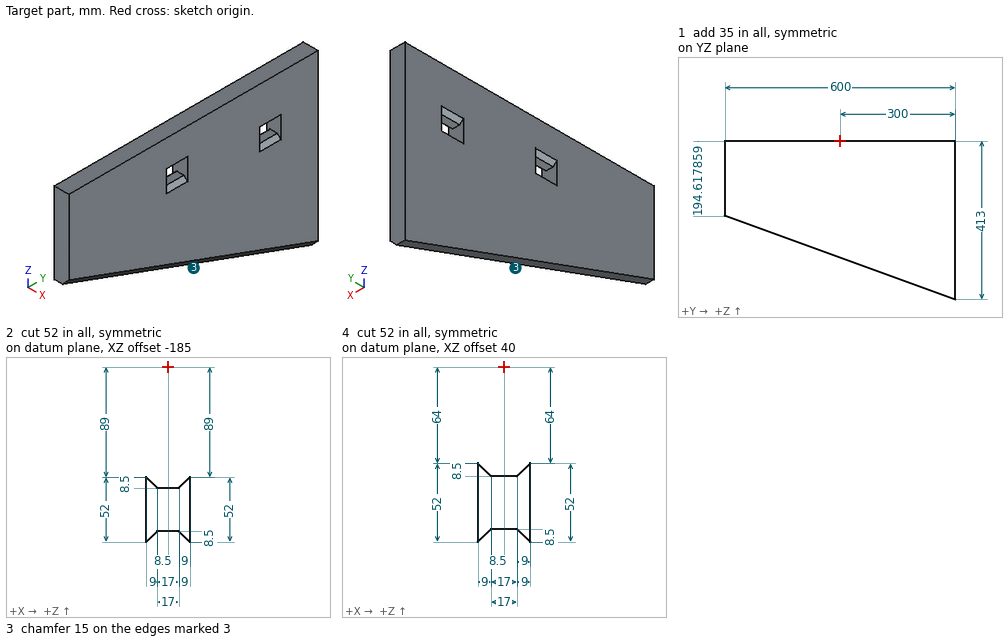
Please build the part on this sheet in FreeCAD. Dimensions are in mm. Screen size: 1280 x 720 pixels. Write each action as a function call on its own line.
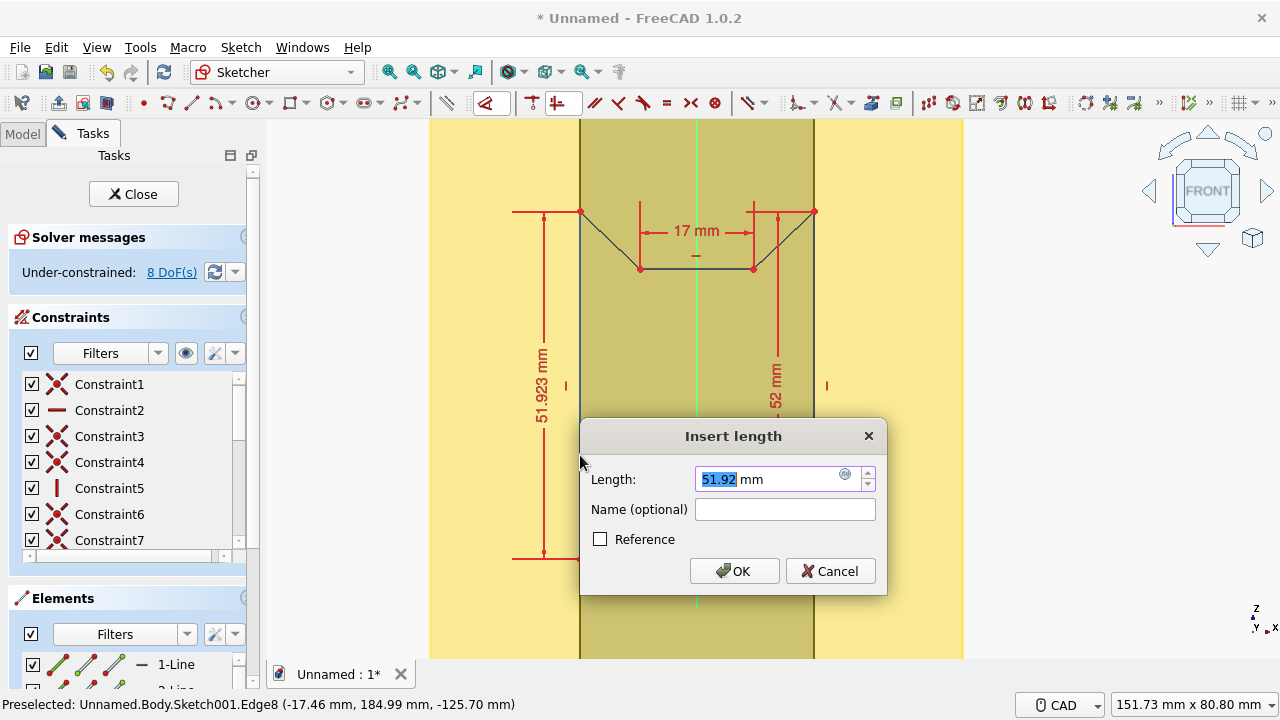
text(52)
key(Return)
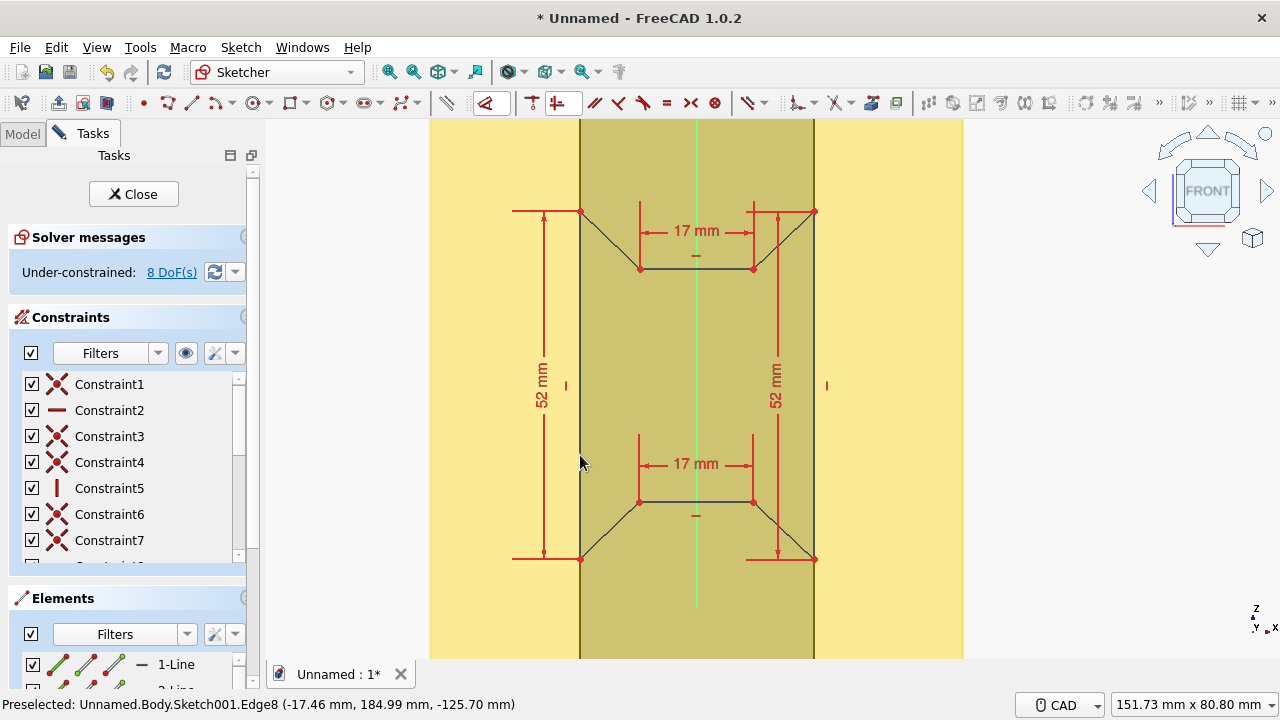
click(598, 229)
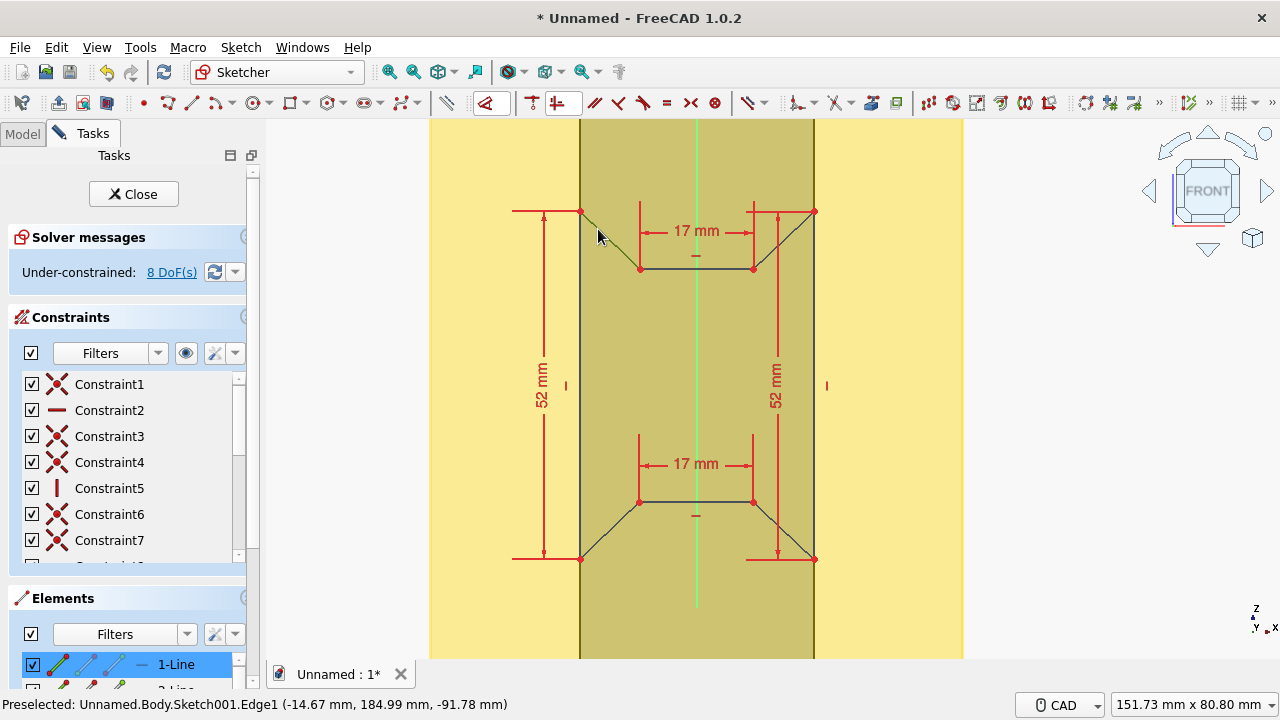
key(l)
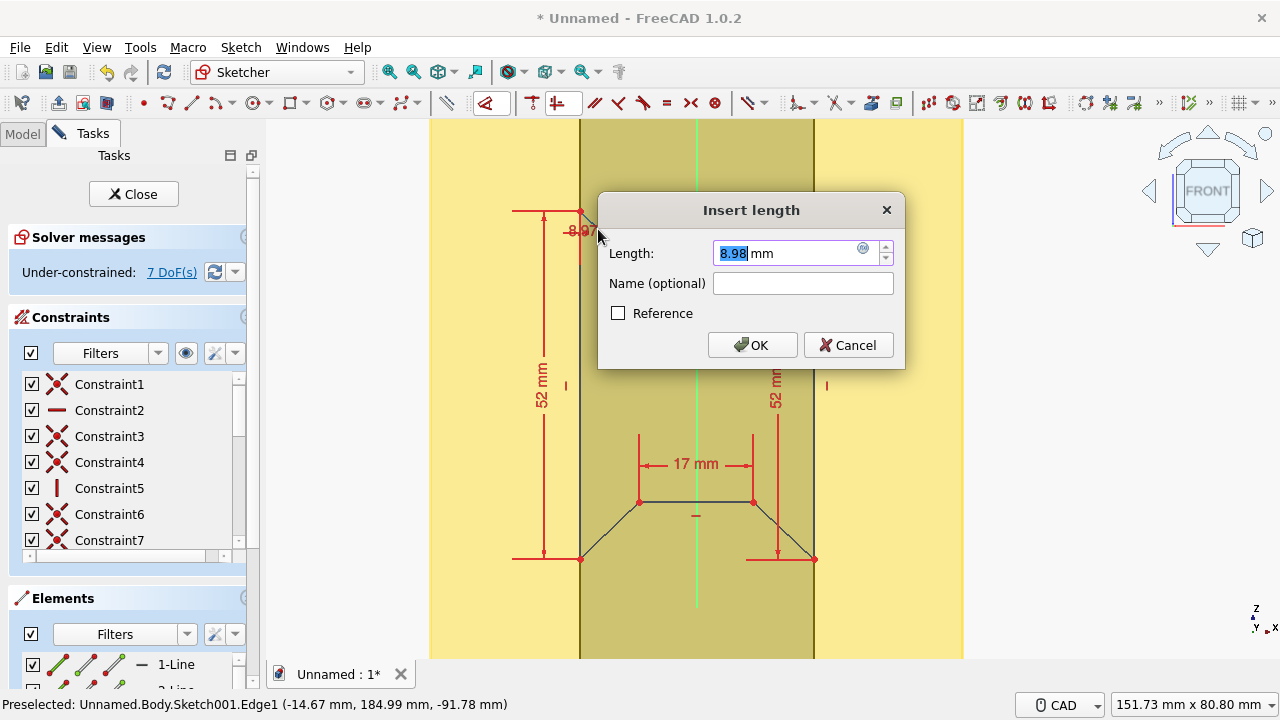
text(9)
key(Return)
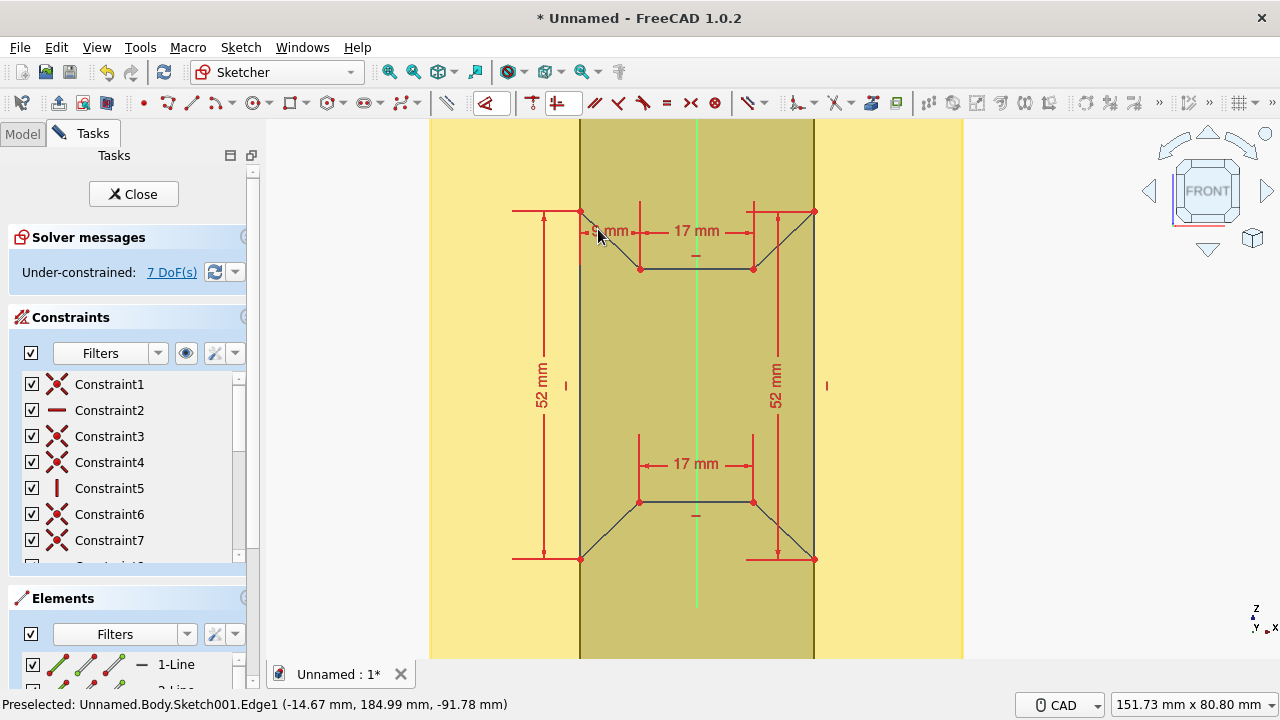
click(772, 252)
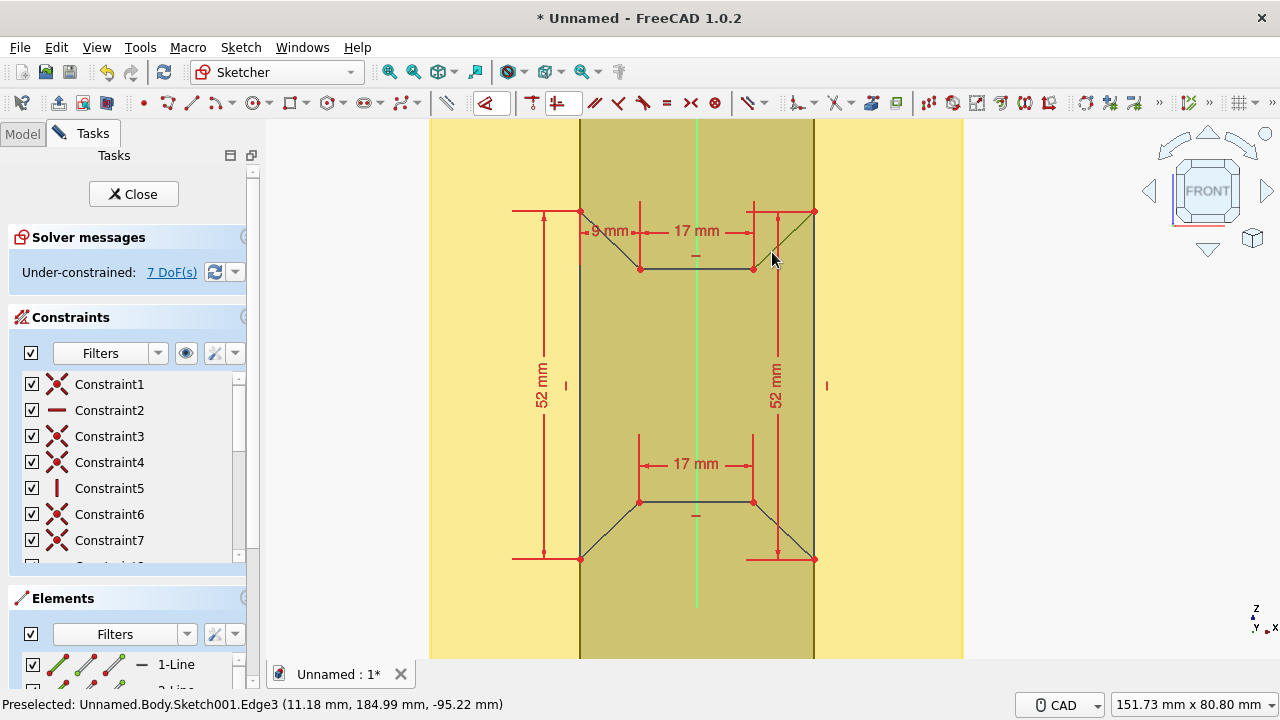
key(l)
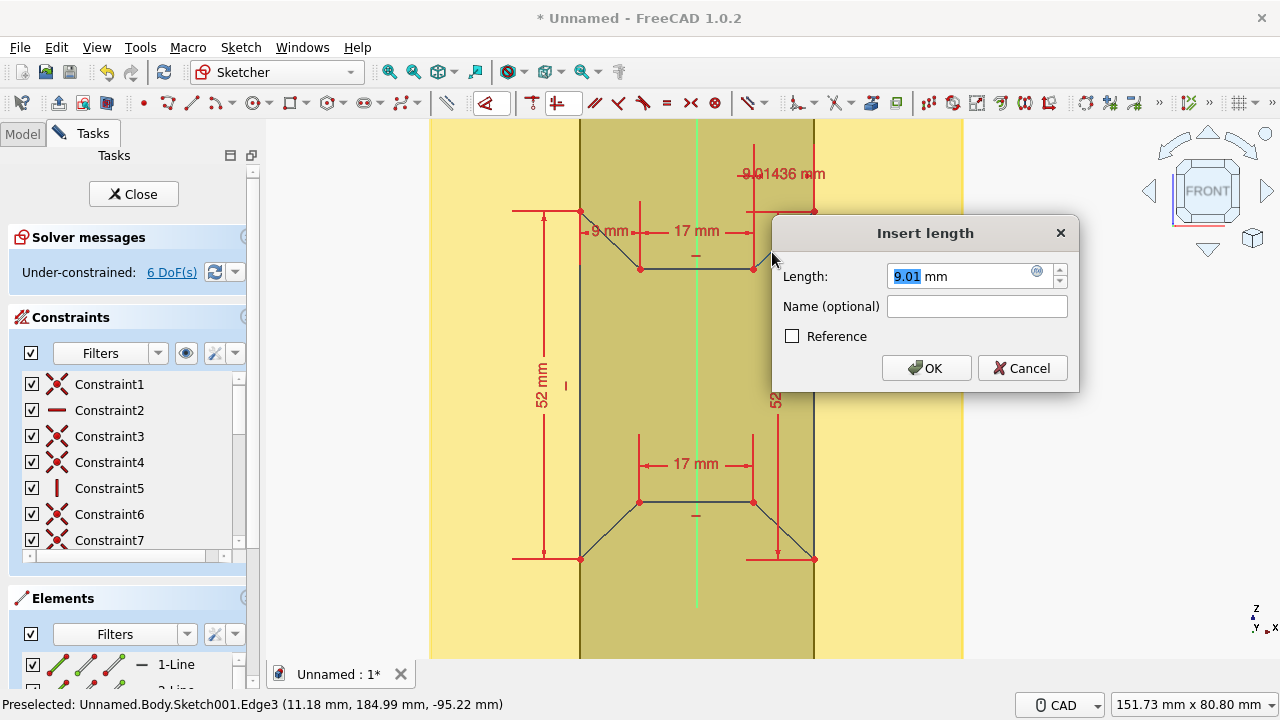
text(9)
key(Return)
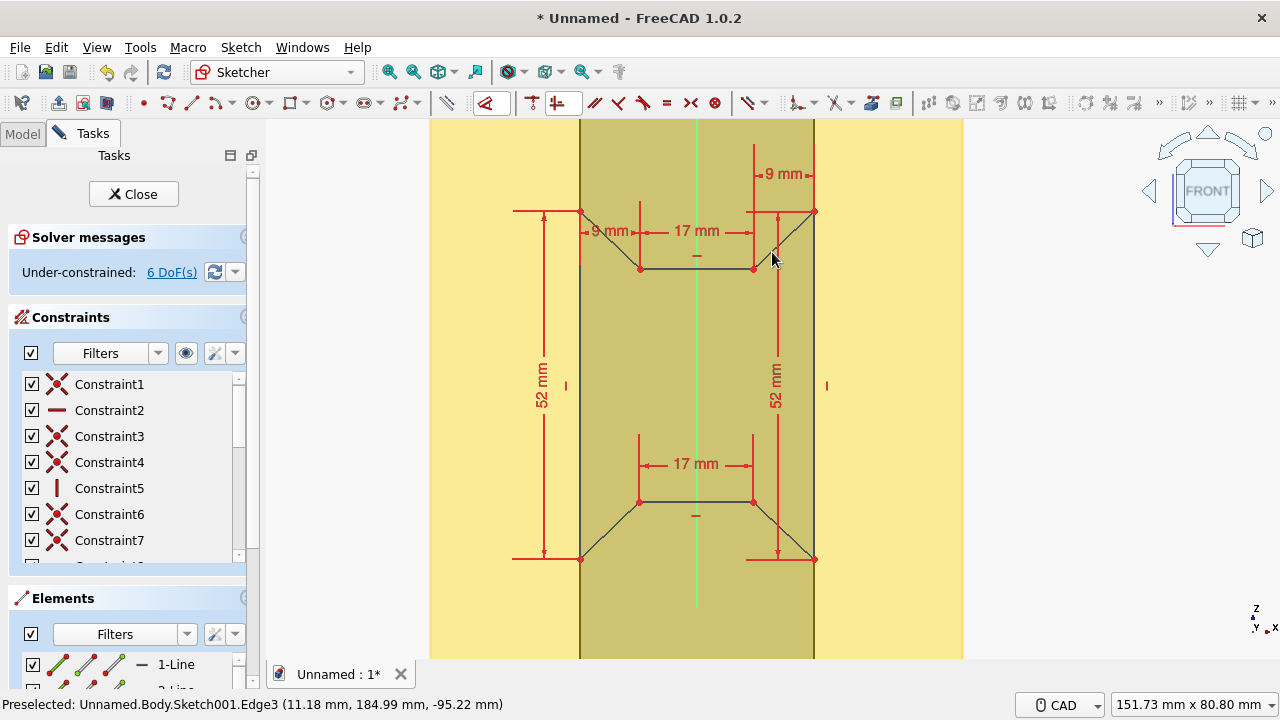
click(796, 542)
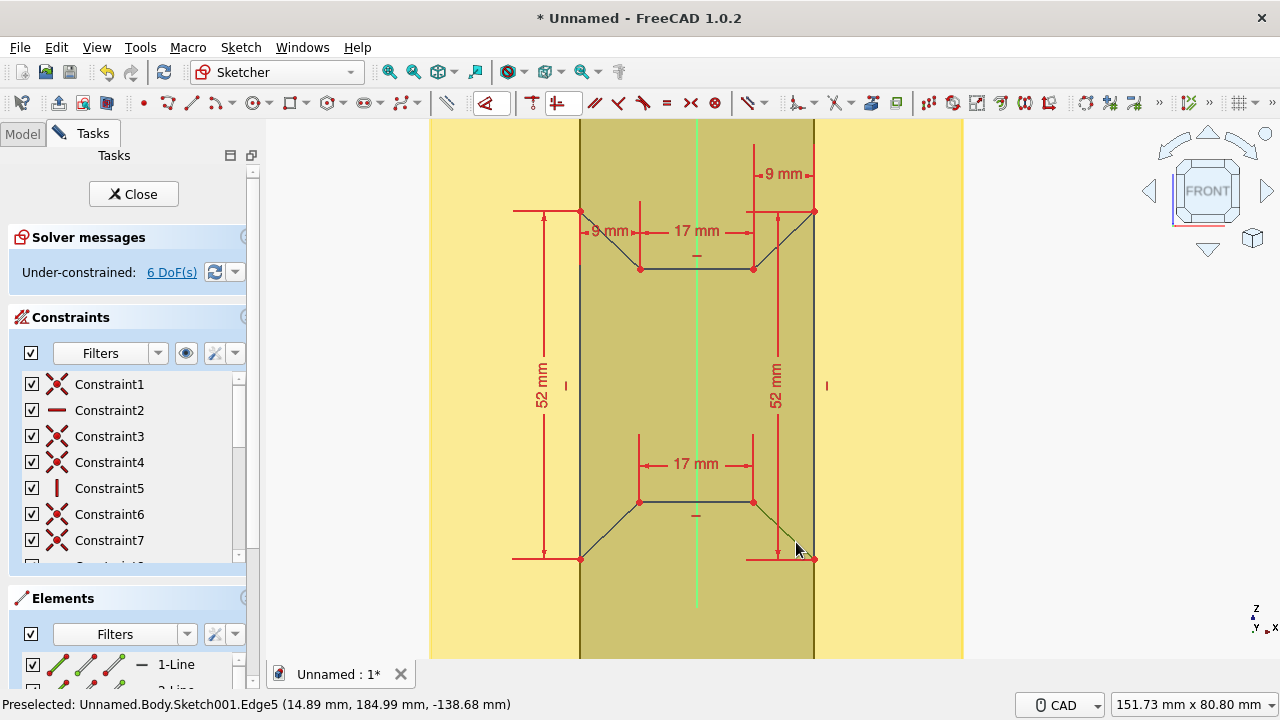
key(l)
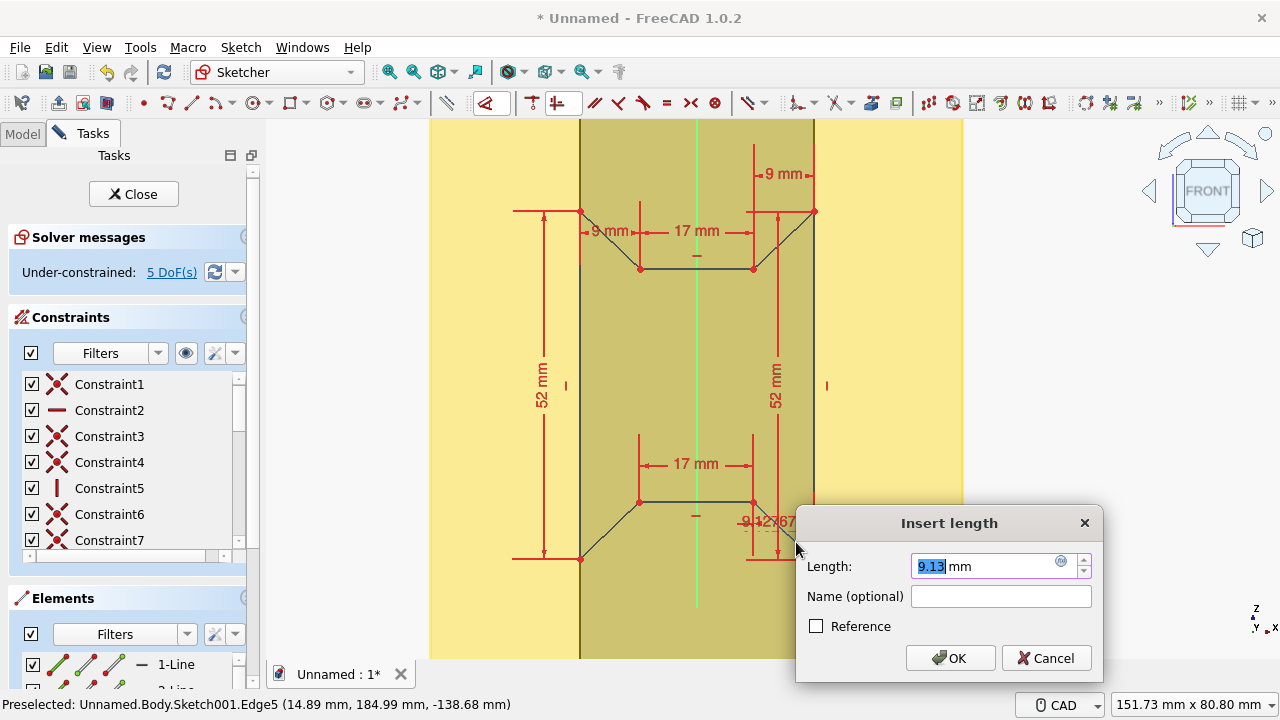
text(9)
key(Return)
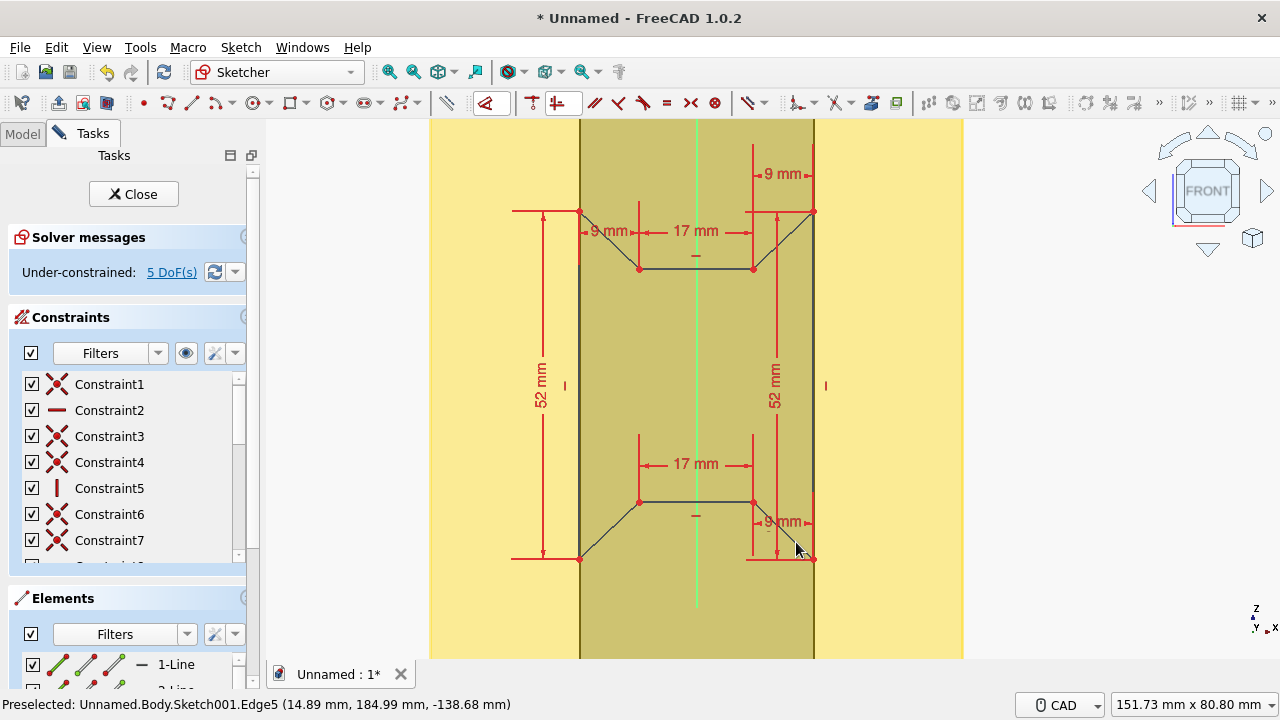
click(579, 211)